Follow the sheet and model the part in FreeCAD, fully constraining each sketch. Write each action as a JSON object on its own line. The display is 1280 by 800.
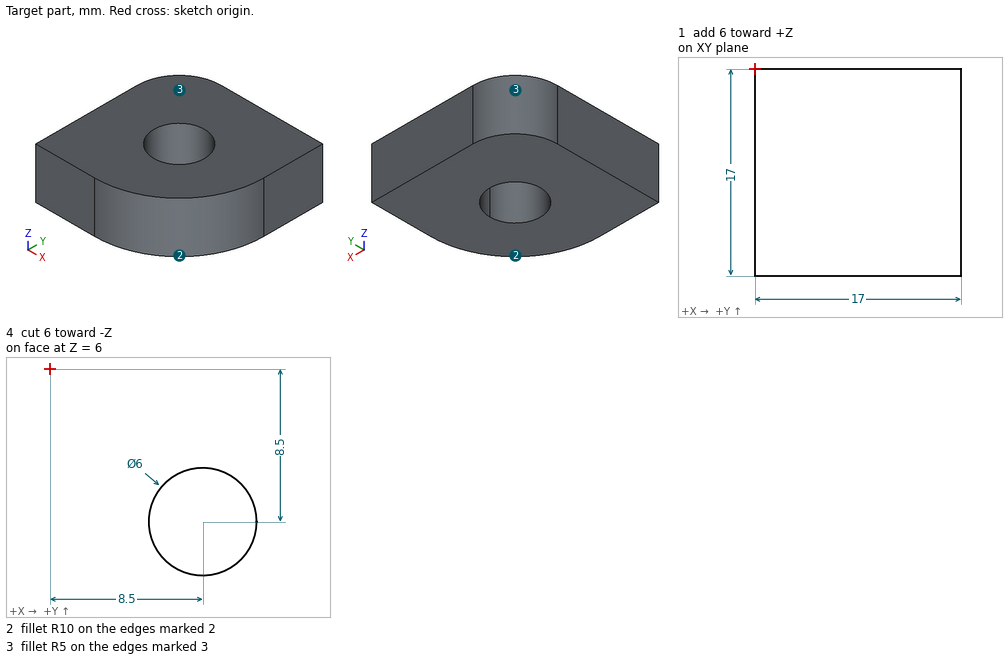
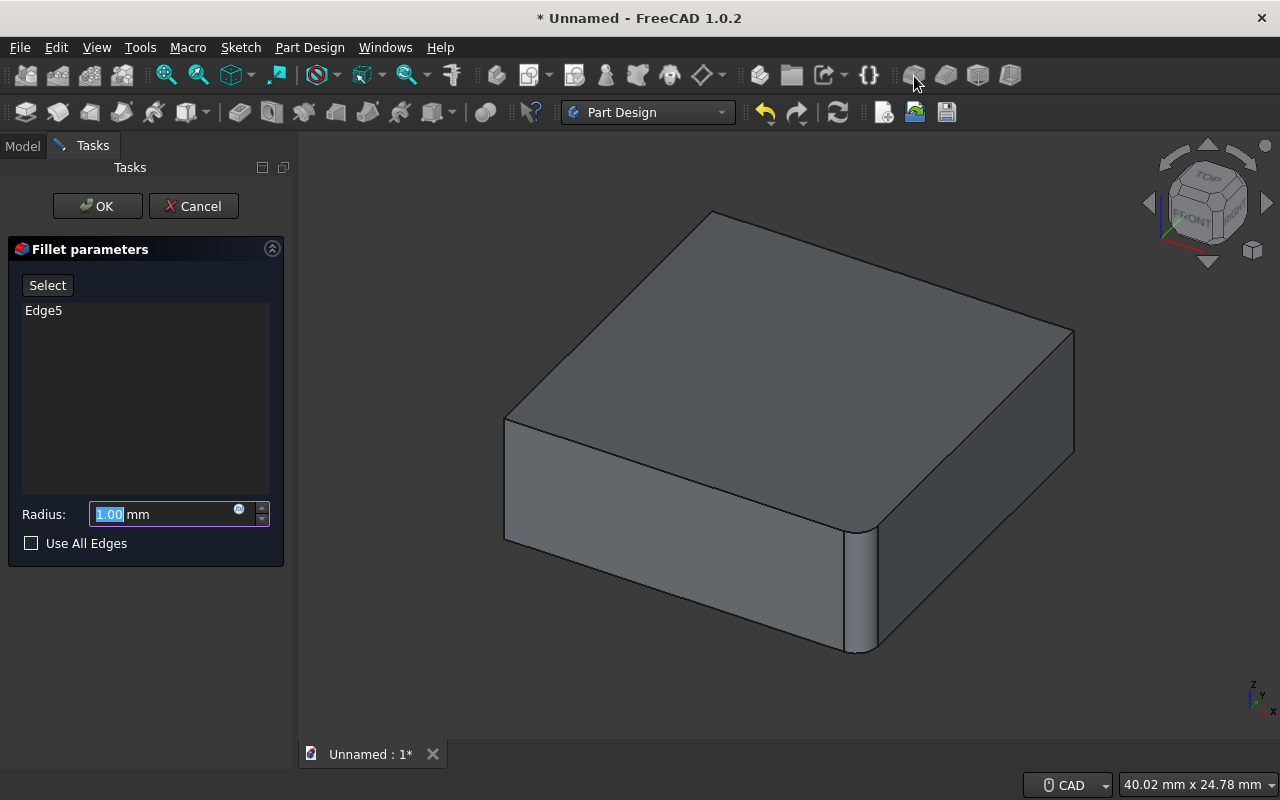
{"action": "type", "text": "10"}
{"action": "key", "text": "Tab"}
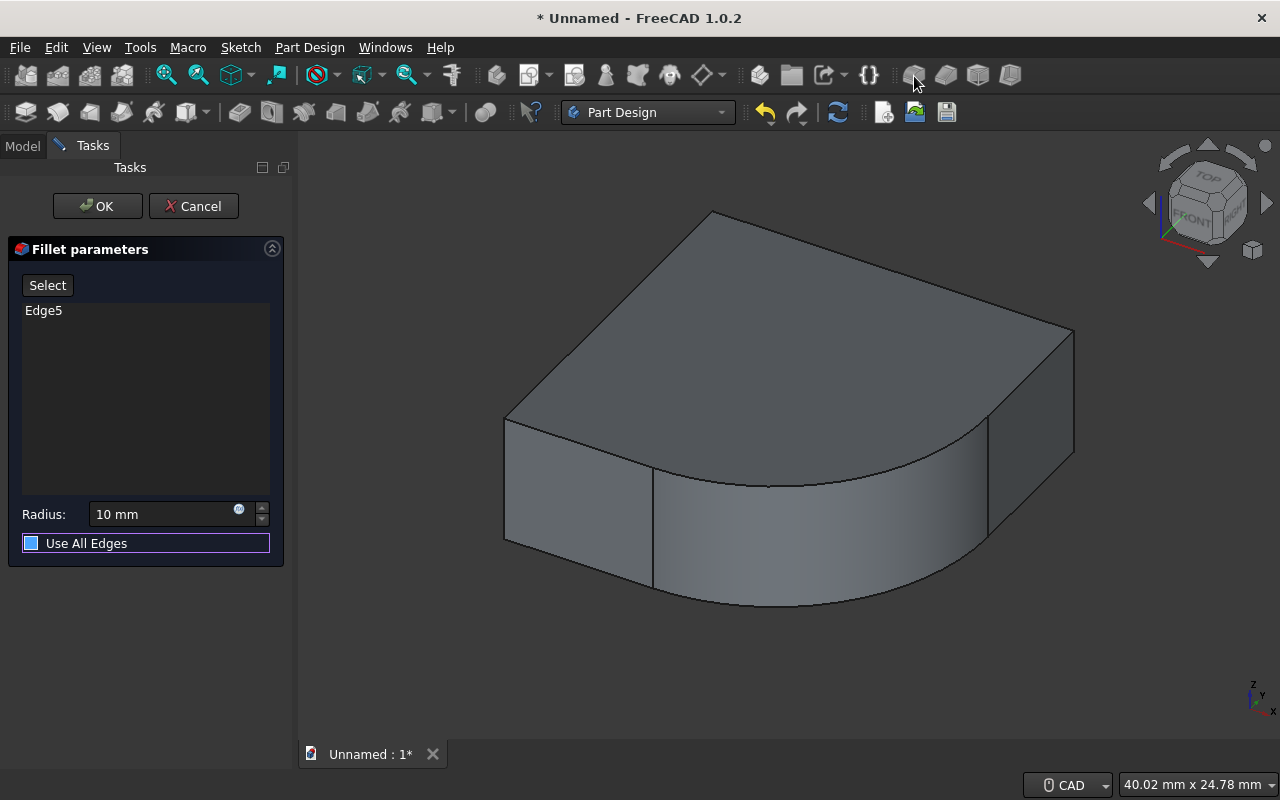
{"action": "left_click", "coordinate": [98, 206]}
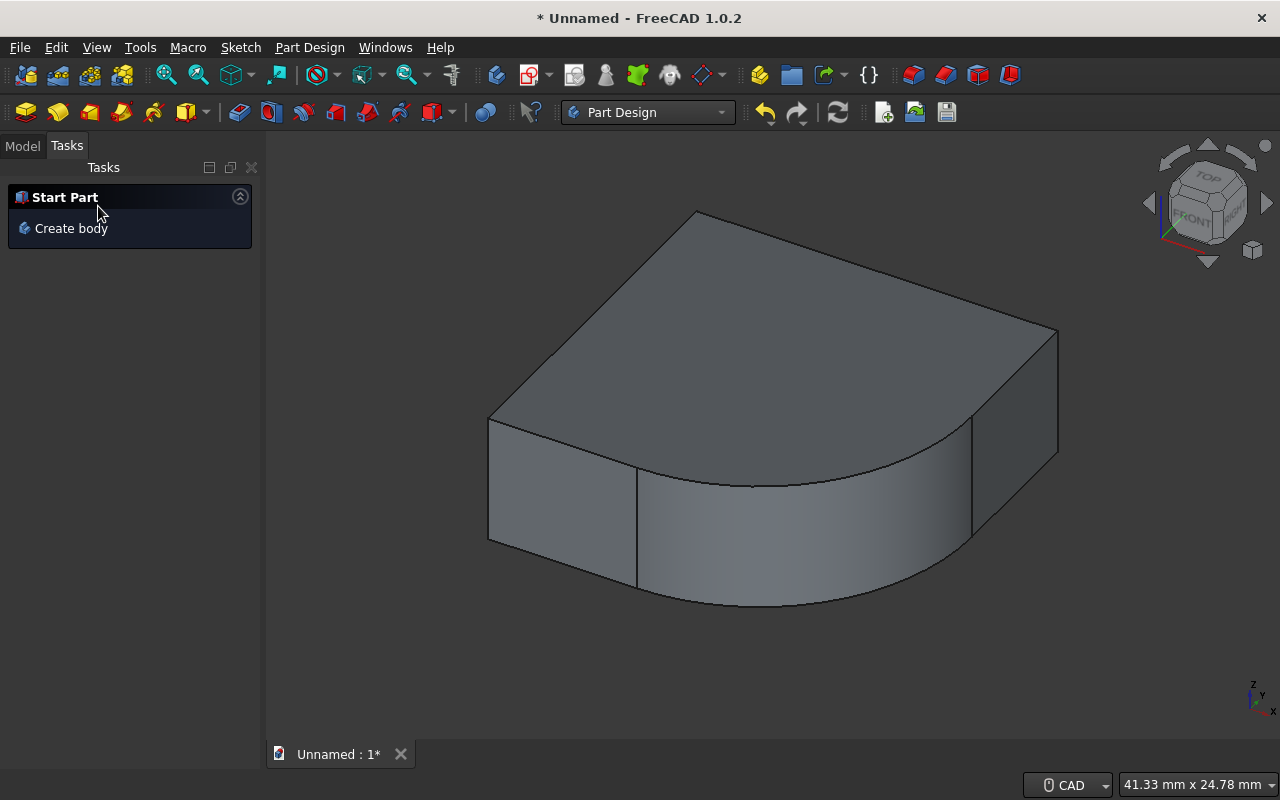
{"action": "key", "text": "0"}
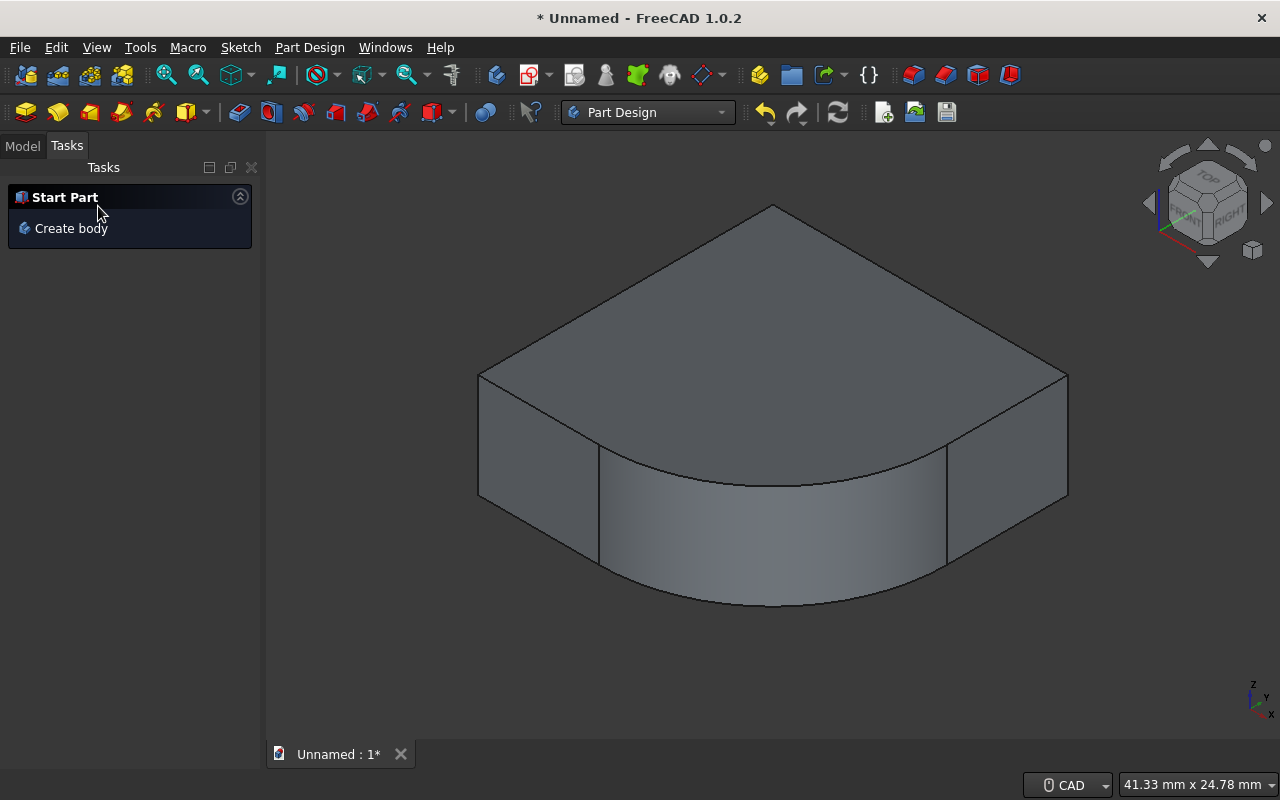
{"action": "key", "text": "2"}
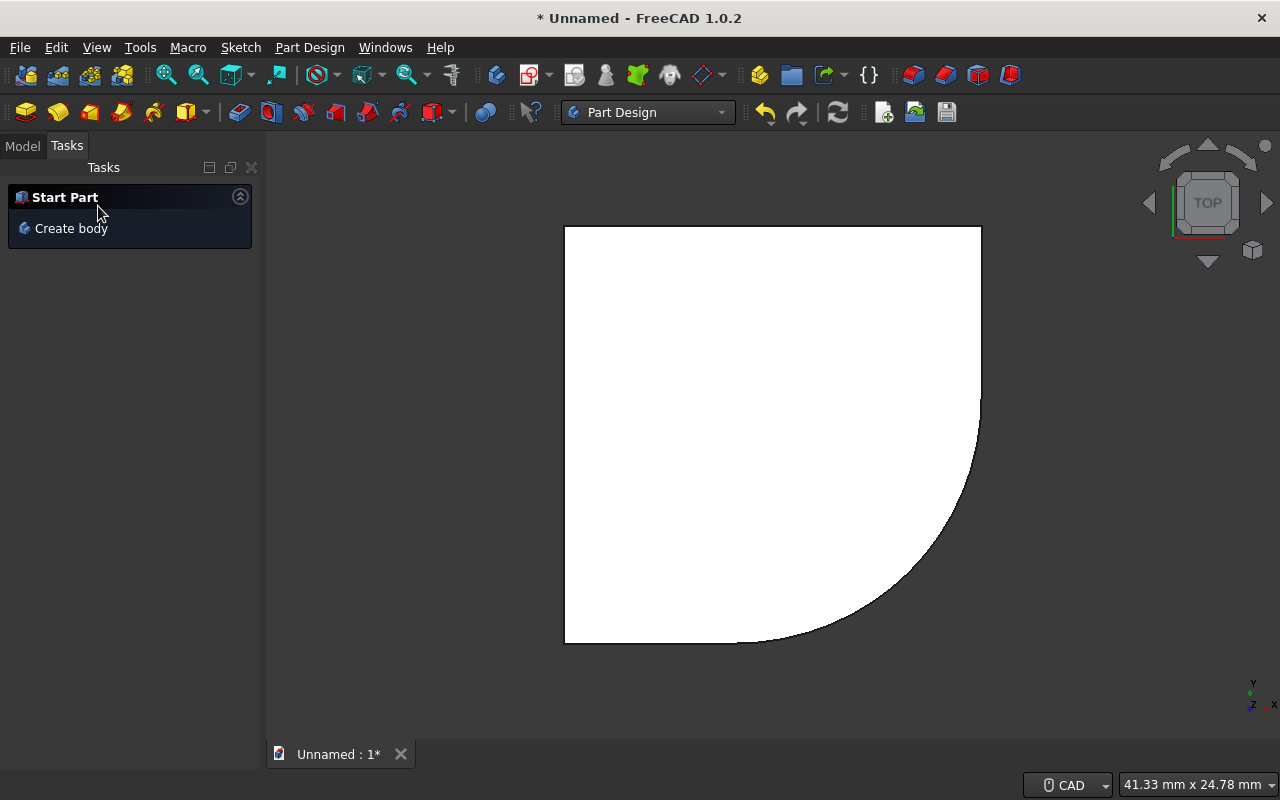
{"action": "key", "text": "1"}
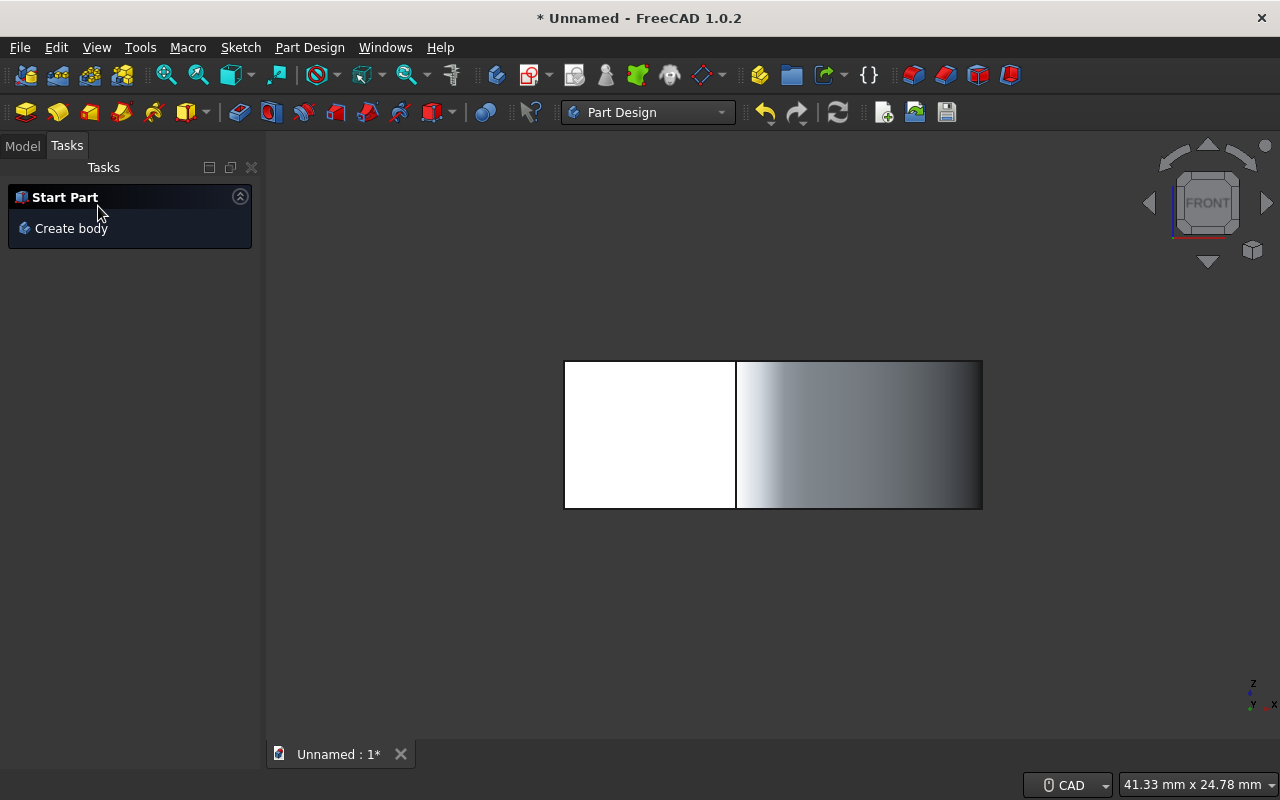
{"action": "left_click", "coordinate": [168, 76]}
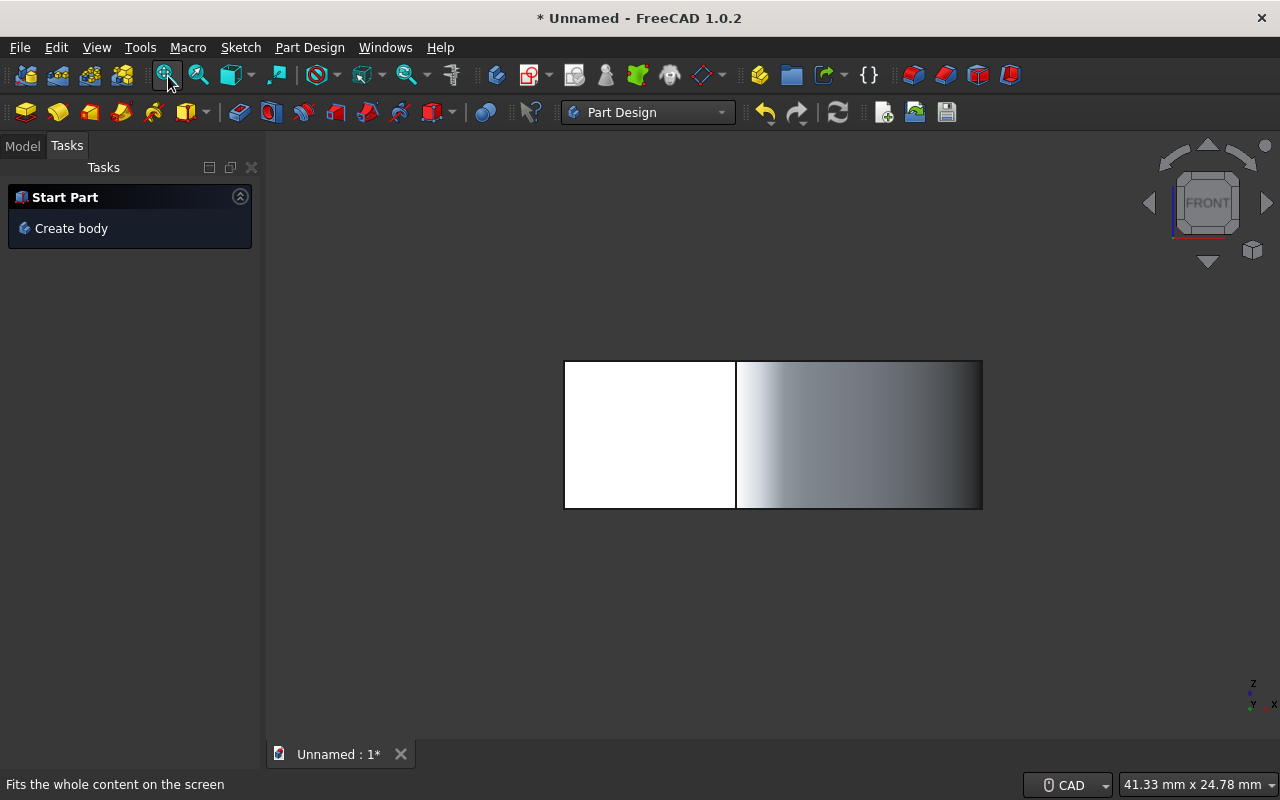
{"action": "key", "text": "3"}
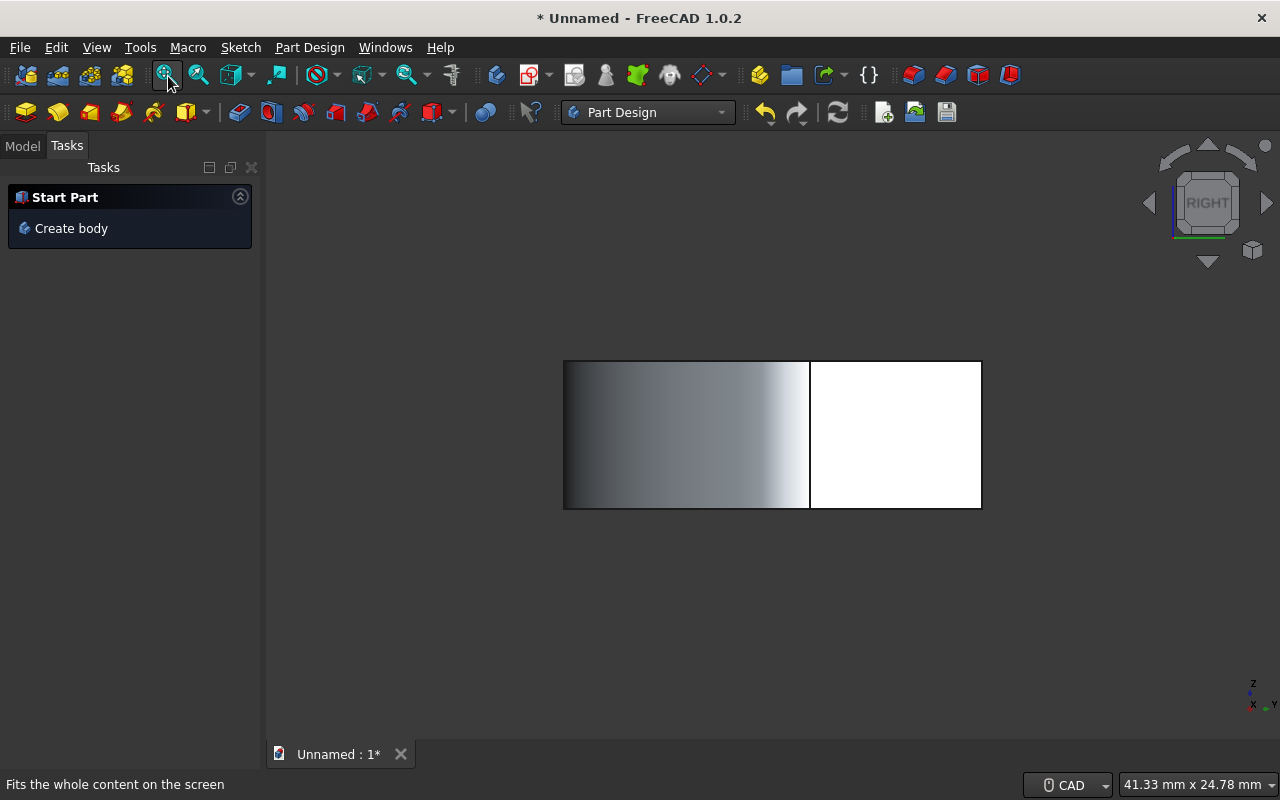
{"action": "left_click", "coordinate": [168, 76]}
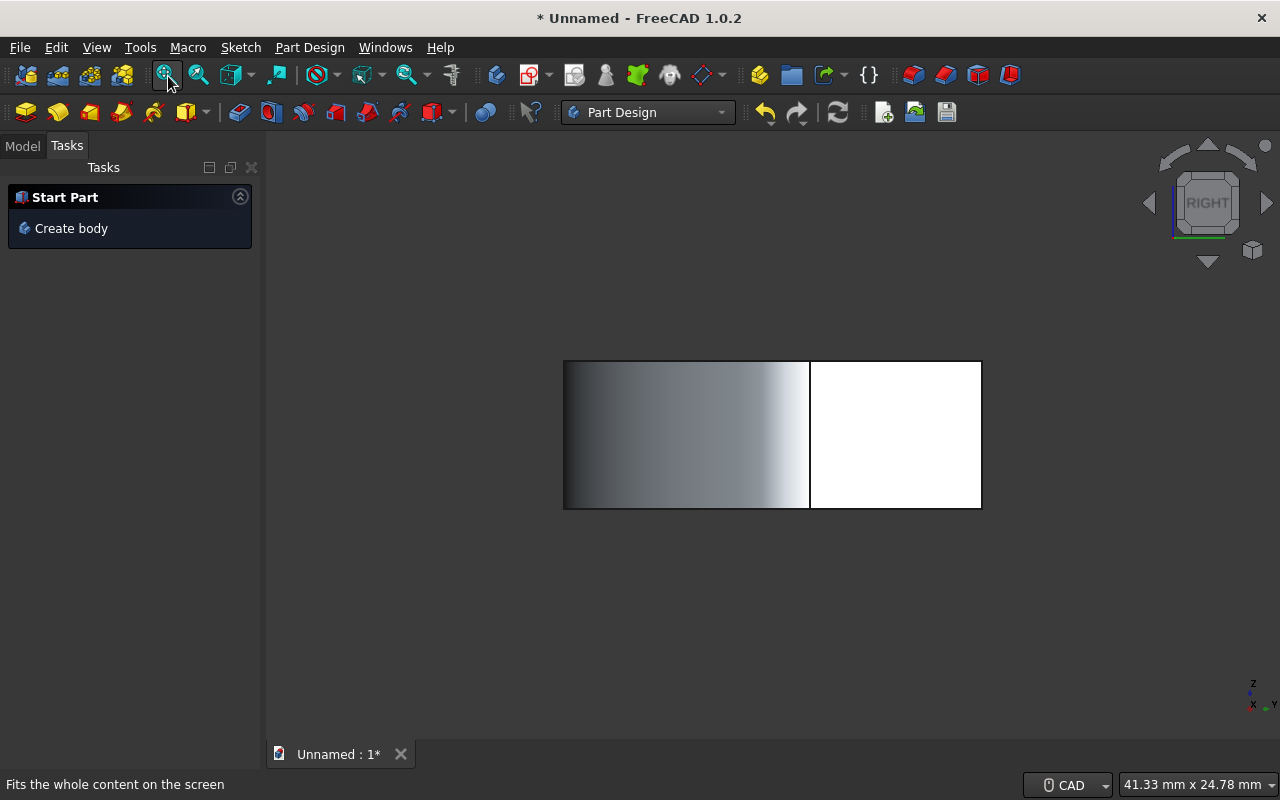
{"action": "key", "text": "5"}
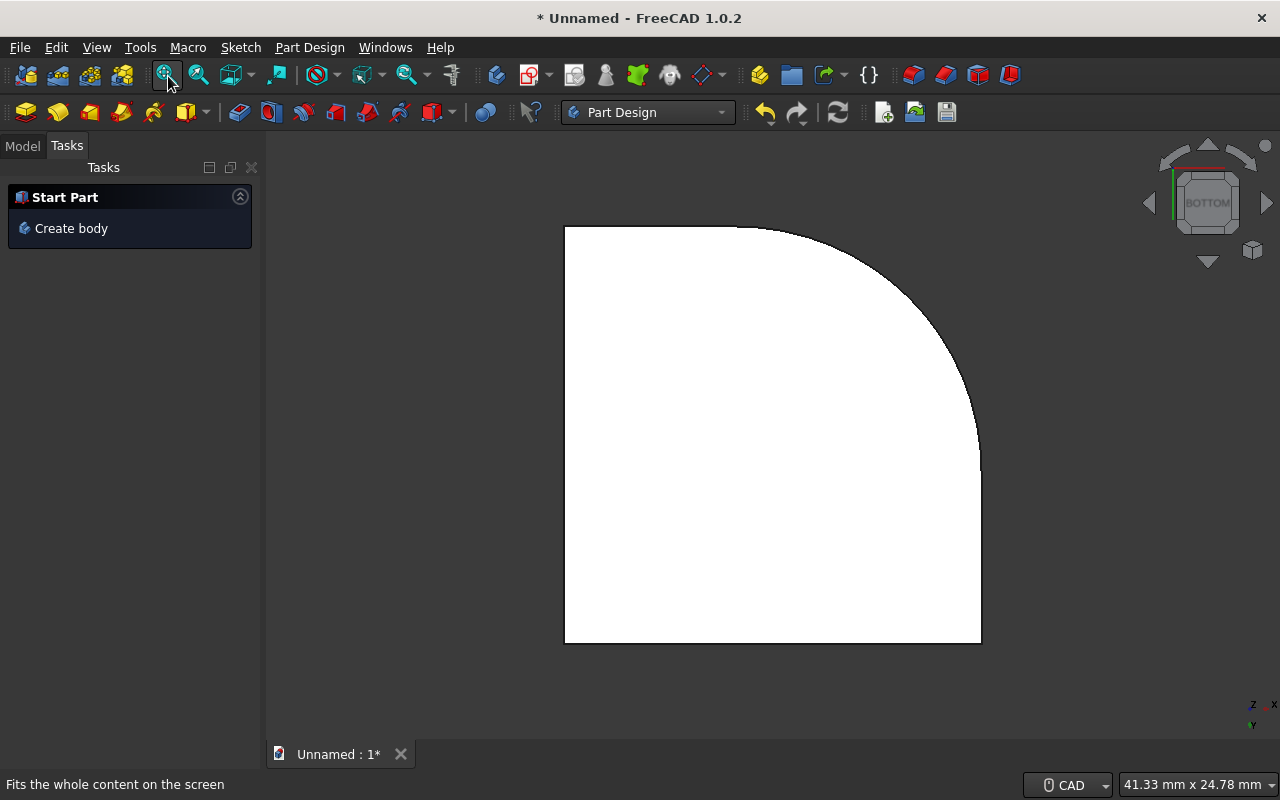
{"action": "key", "text": "4"}